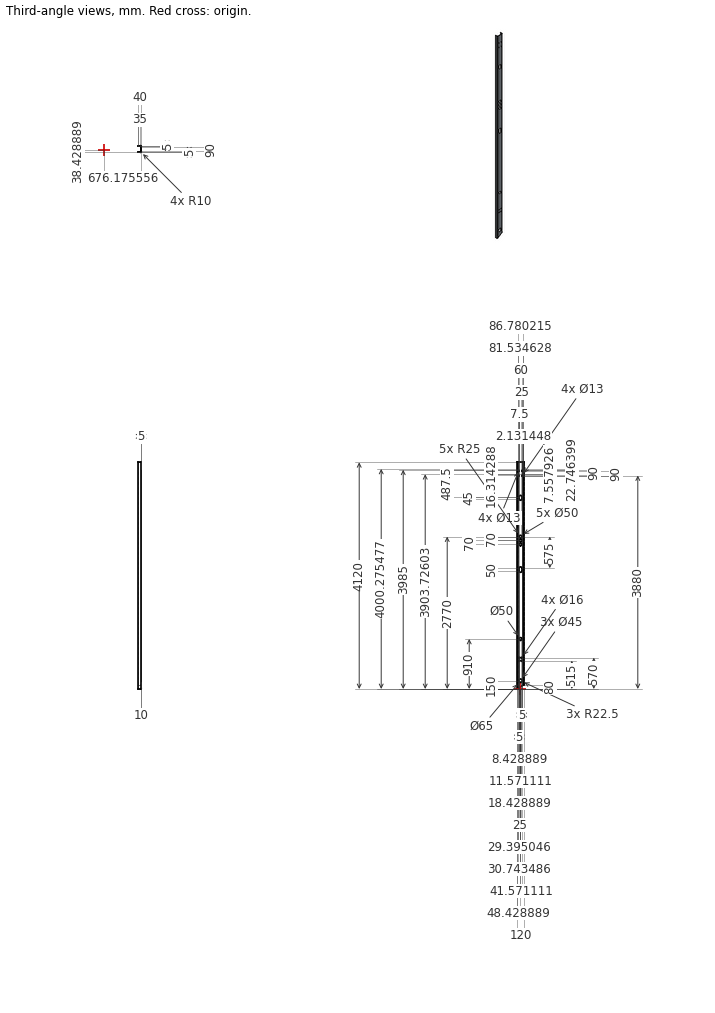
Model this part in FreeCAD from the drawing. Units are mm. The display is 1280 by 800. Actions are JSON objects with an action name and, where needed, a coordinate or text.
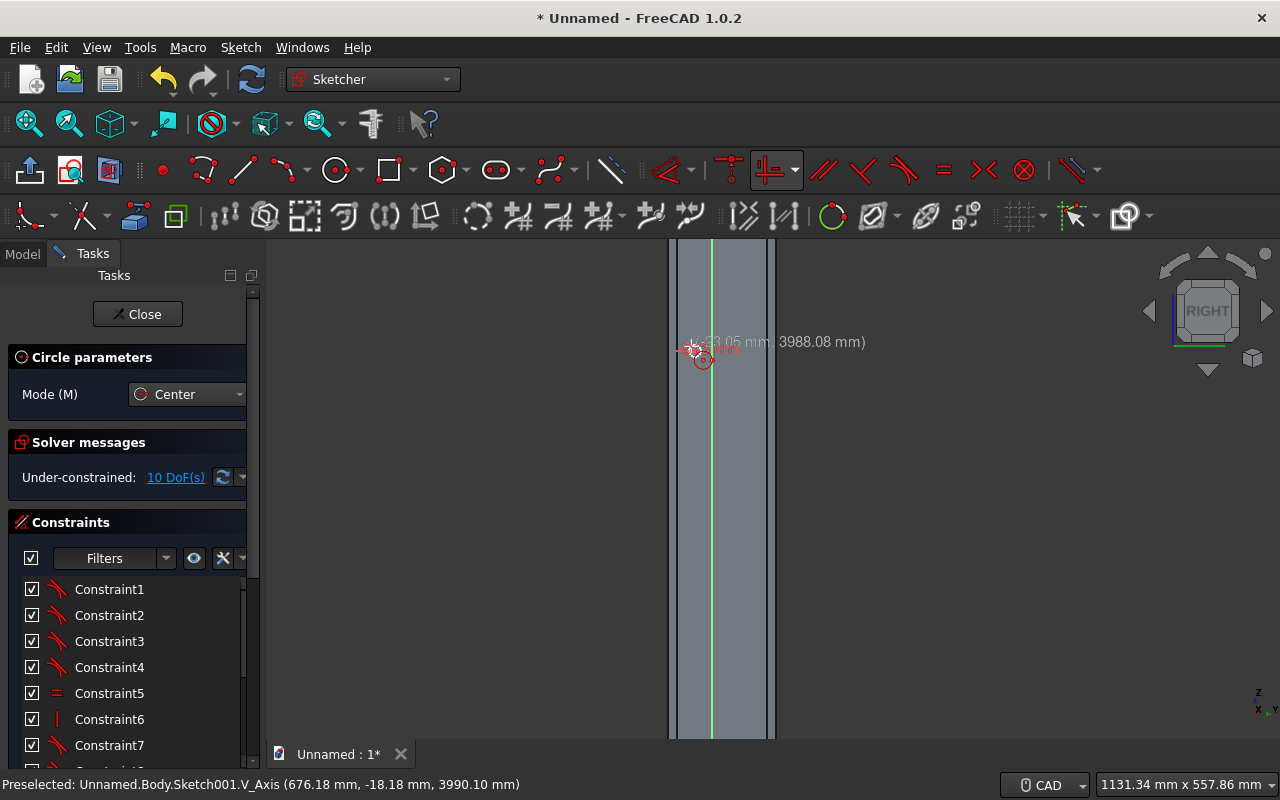
{"action": "scroll", "coordinate": [749, 350], "scroll_direction": "up", "scroll_amount": 7}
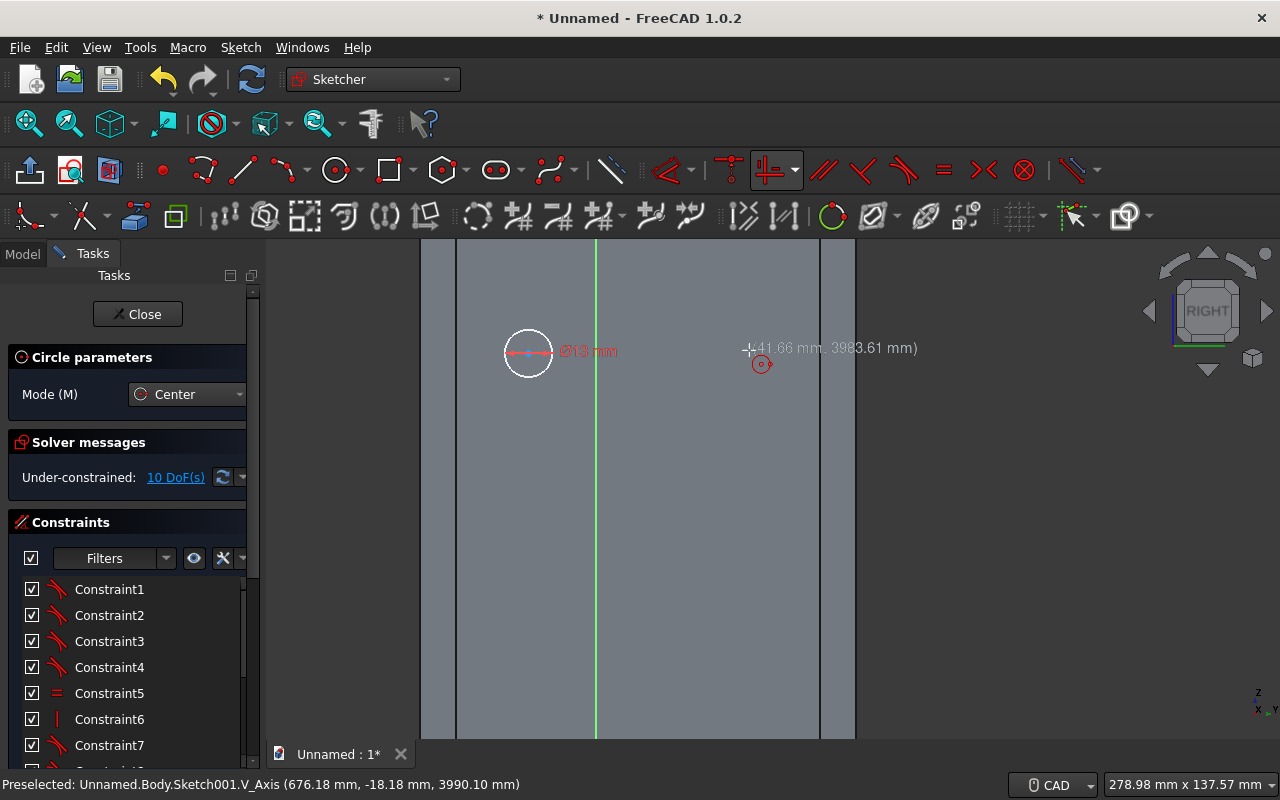
{"action": "scroll", "coordinate": [704, 489], "scroll_direction": "down", "scroll_amount": 15}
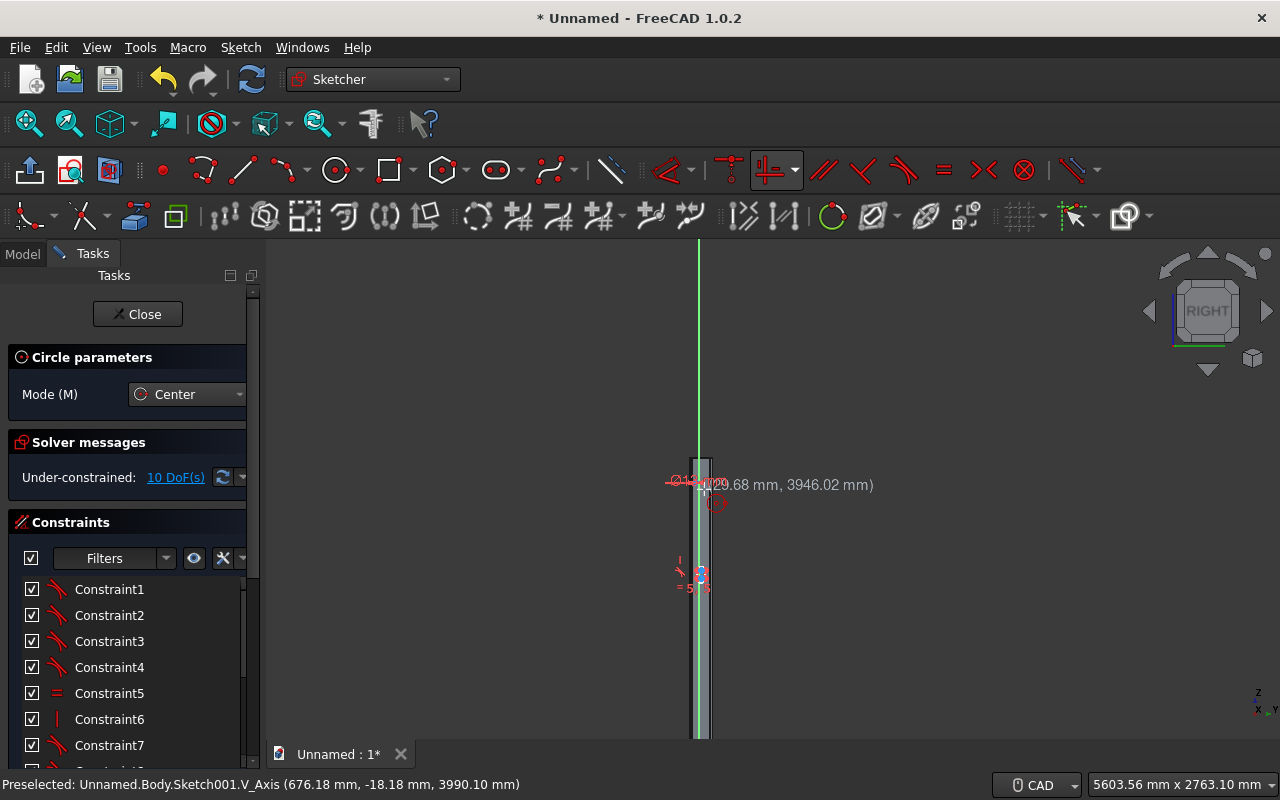
{"action": "scroll", "coordinate": [706, 283], "scroll_direction": "down", "scroll_amount": 5}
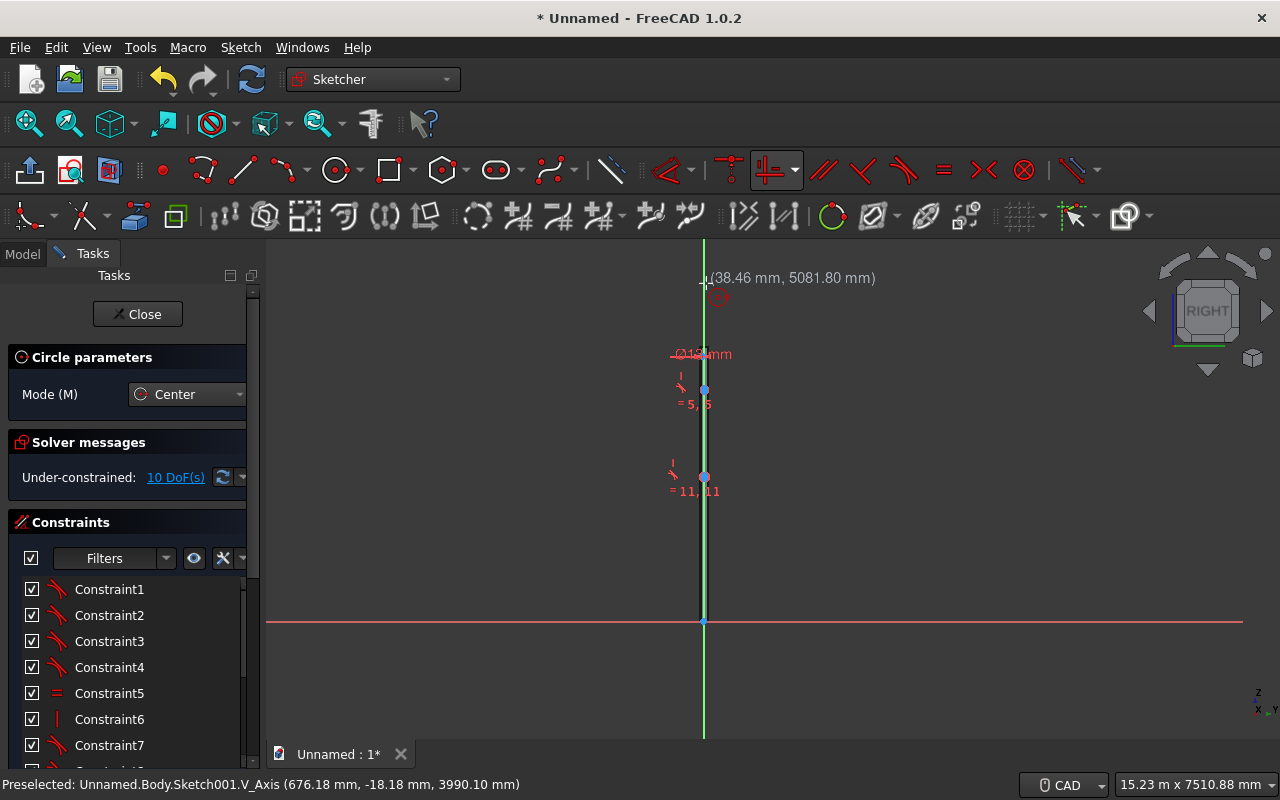
{"action": "scroll", "coordinate": [706, 356], "scroll_direction": "up", "scroll_amount": 9}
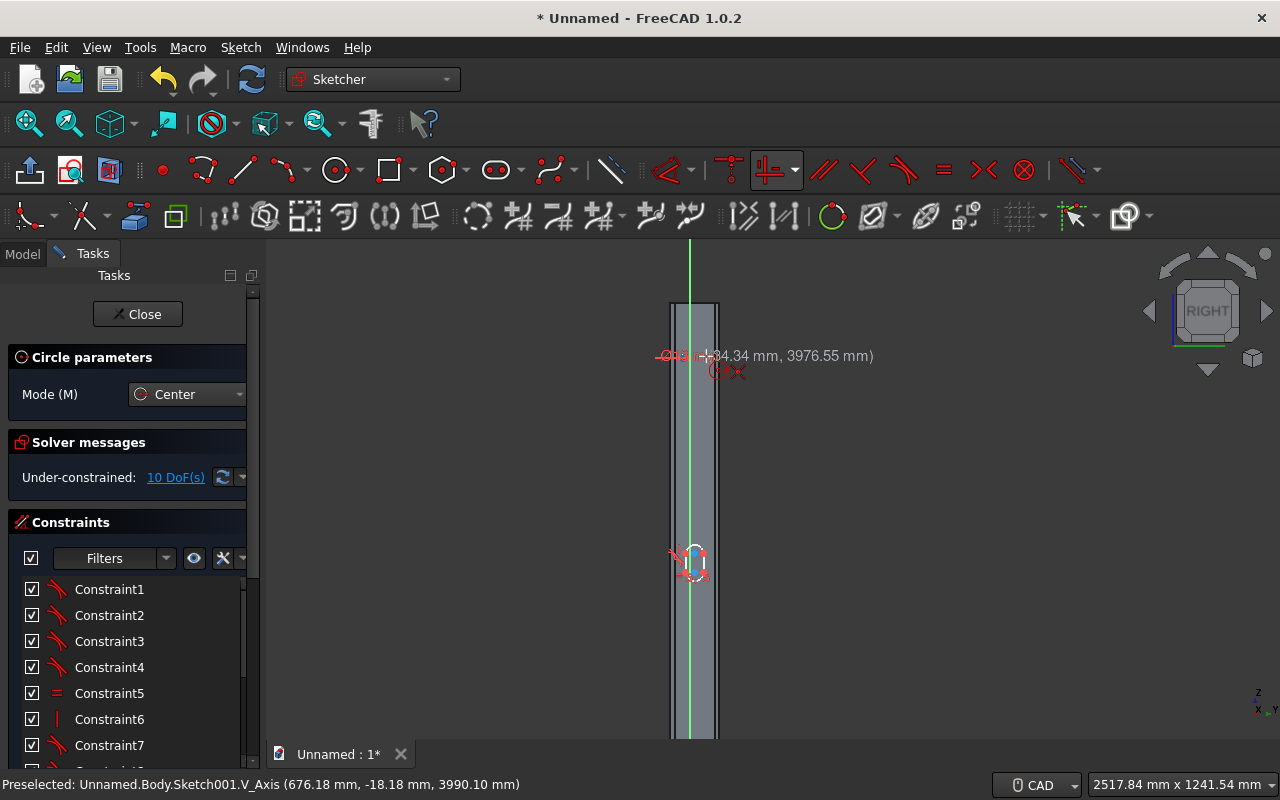
{"action": "left_click", "coordinate": [707, 357]}
{"action": "mouse_move", "coordinate": [709, 356]}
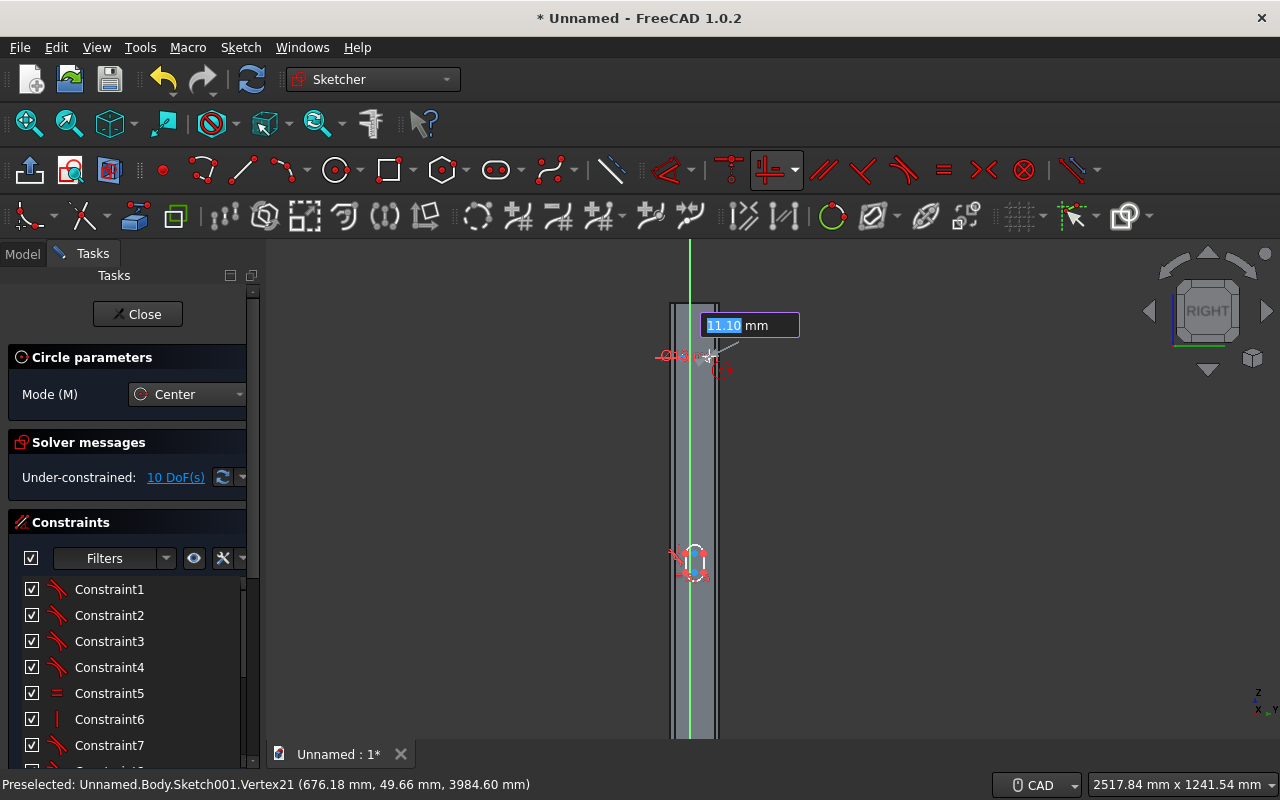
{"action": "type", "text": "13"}
{"action": "key", "text": "Return"}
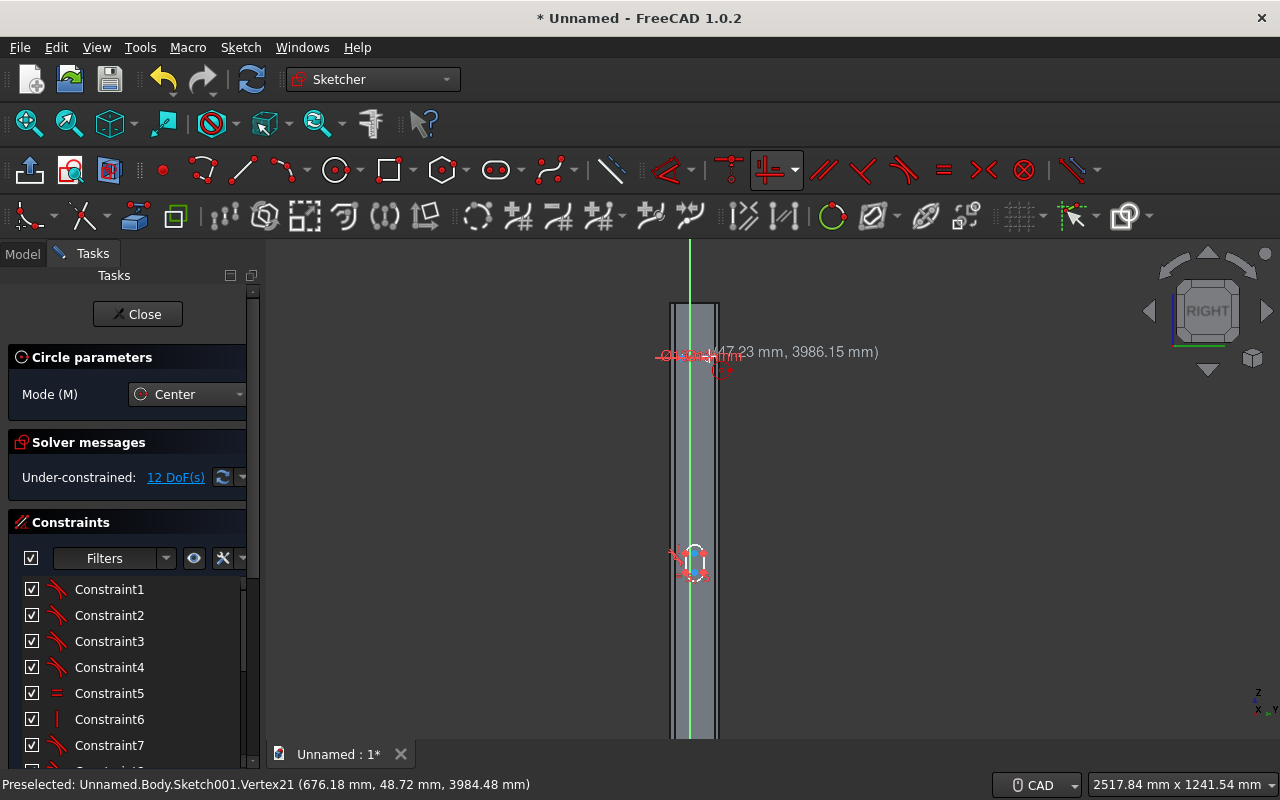
{"action": "scroll", "coordinate": [707, 394], "scroll_direction": "up", "scroll_amount": 11}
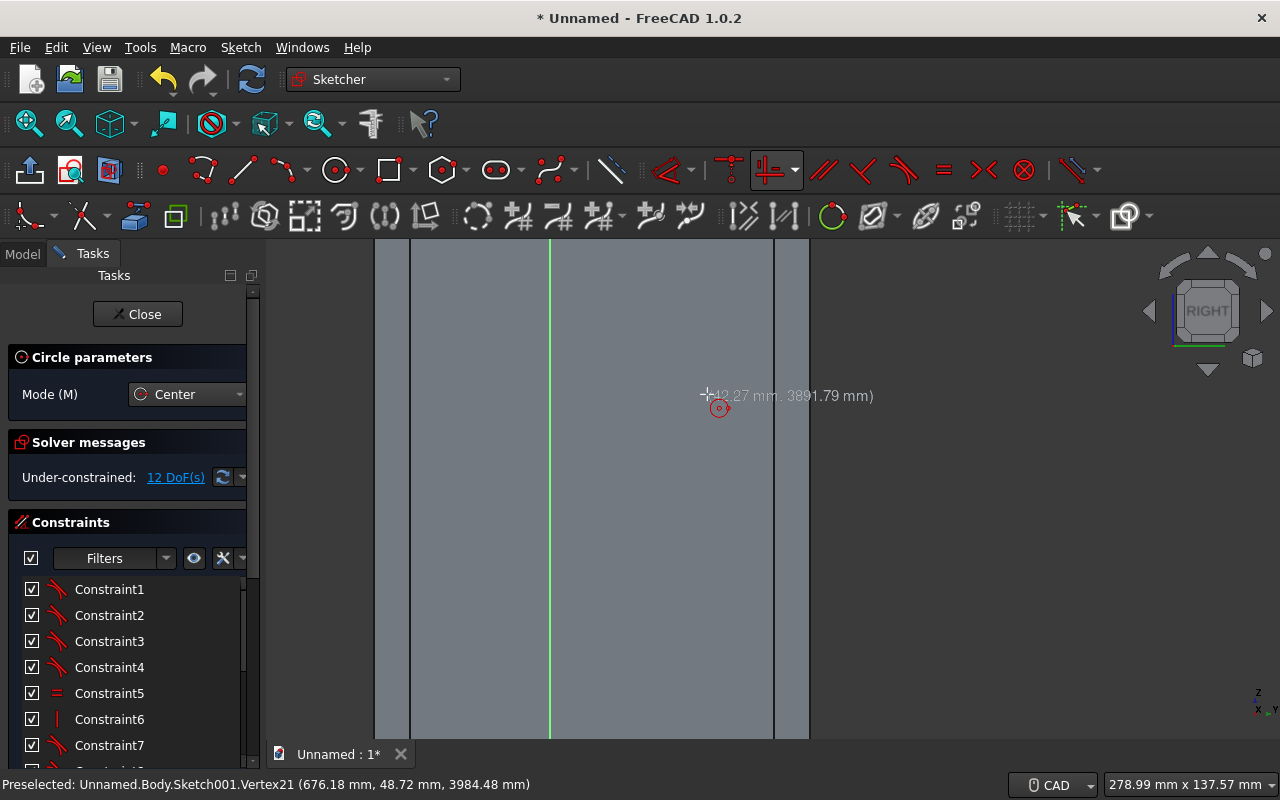
{"action": "scroll", "coordinate": [704, 489], "scroll_direction": "down", "scroll_amount": 15}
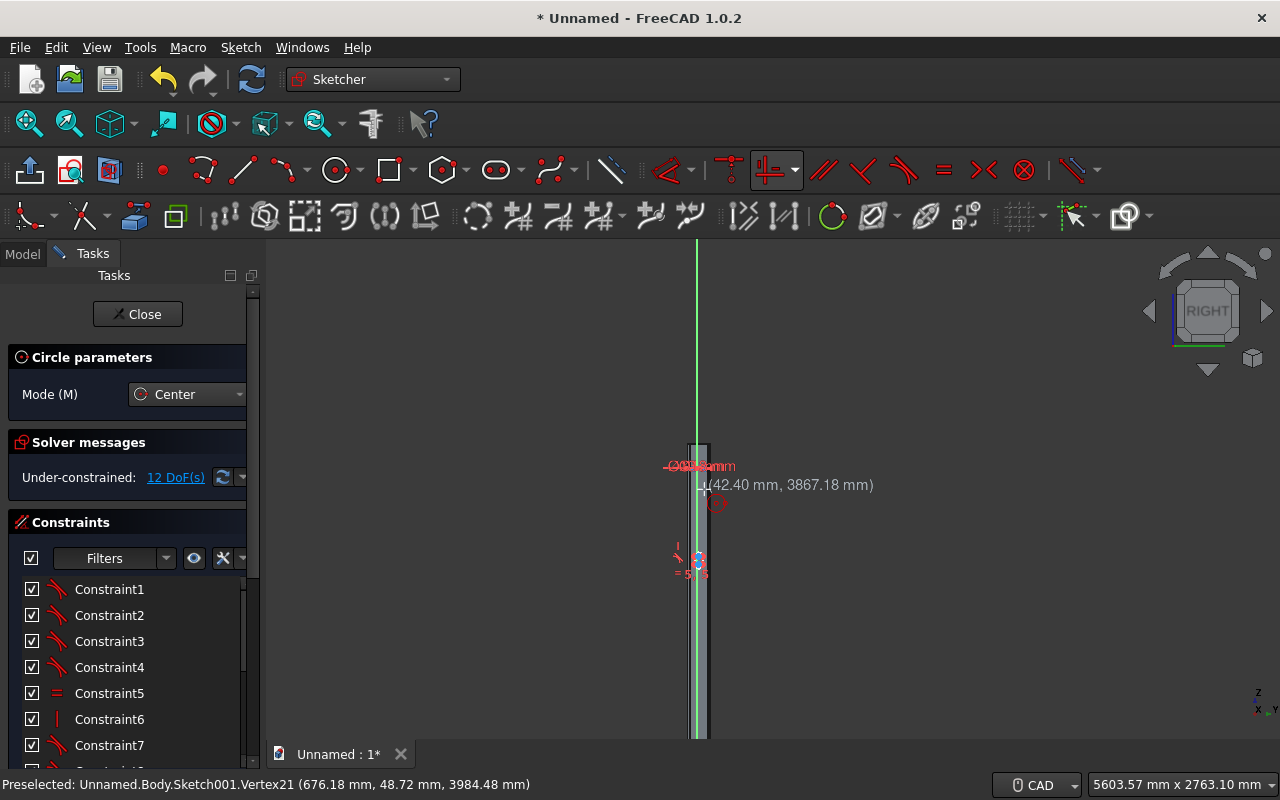
{"action": "scroll", "coordinate": [709, 267], "scroll_direction": "down", "scroll_amount": 4}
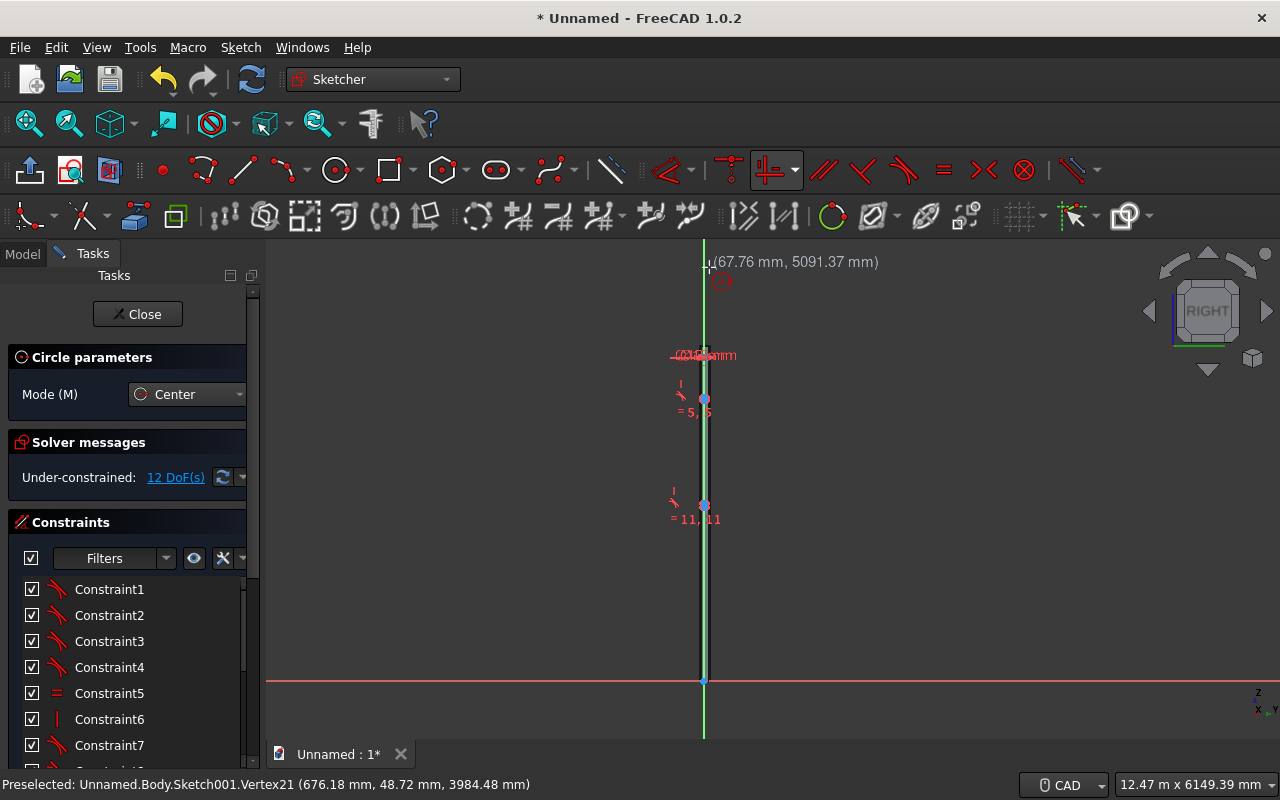
{"action": "scroll", "coordinate": [707, 365], "scroll_direction": "up", "scroll_amount": 8}